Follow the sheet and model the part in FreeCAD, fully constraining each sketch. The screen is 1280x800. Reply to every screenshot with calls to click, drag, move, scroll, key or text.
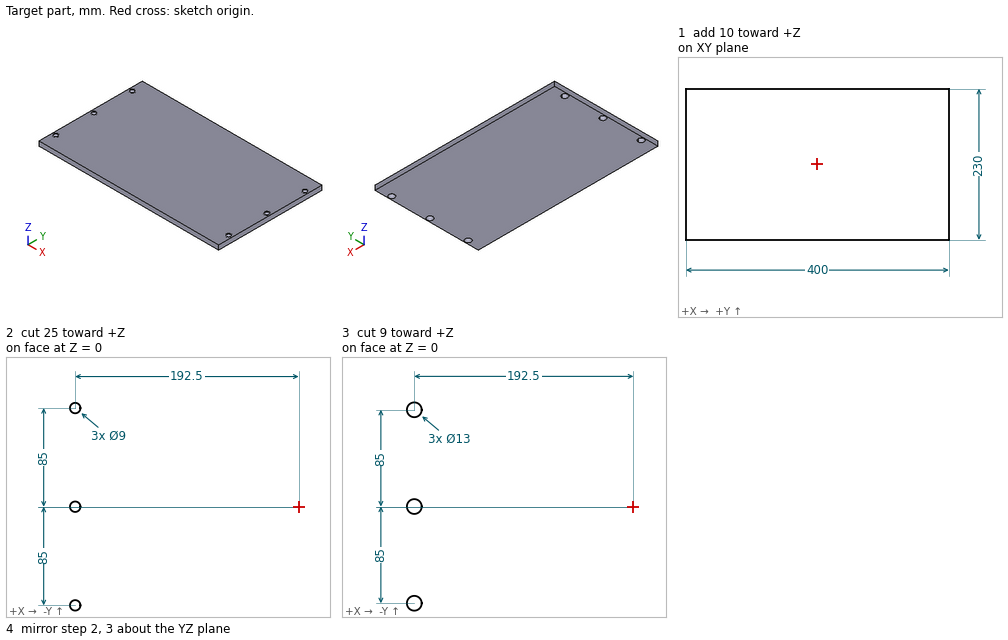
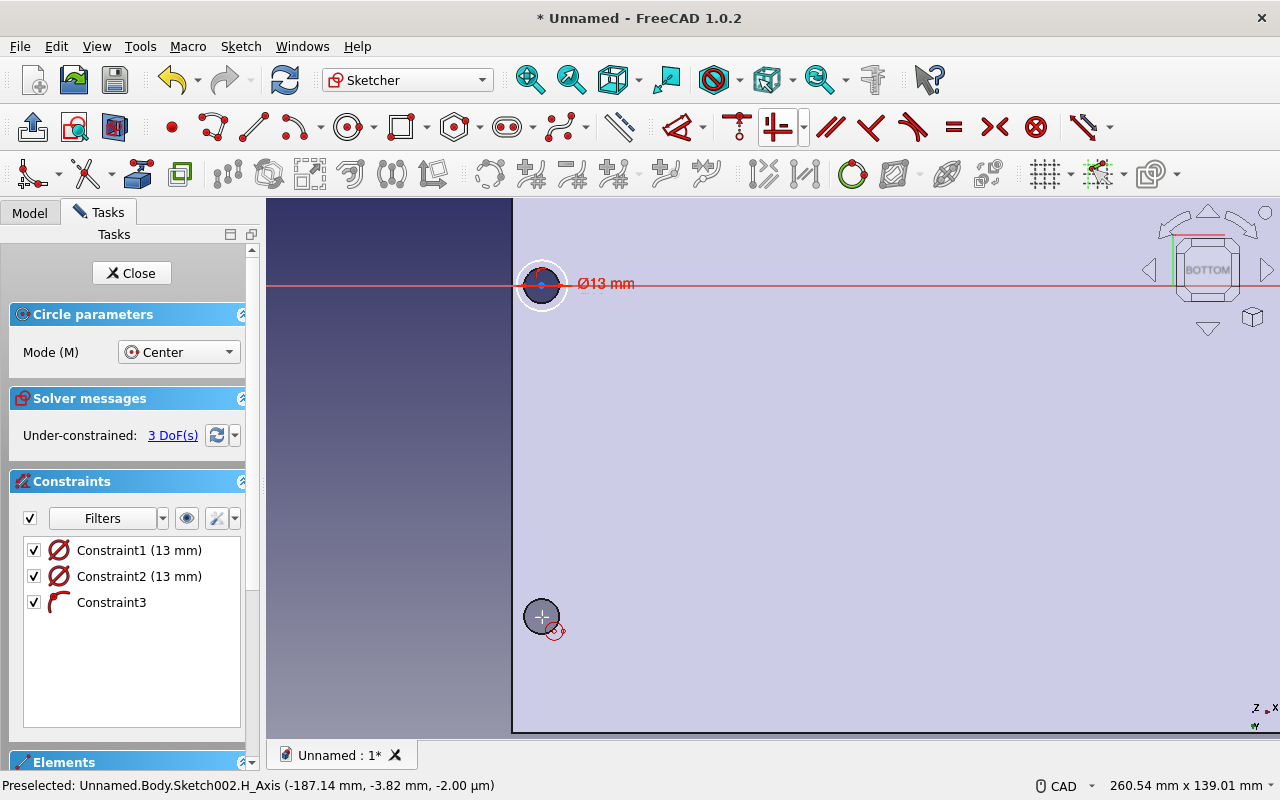
click(542, 616)
move(559, 599)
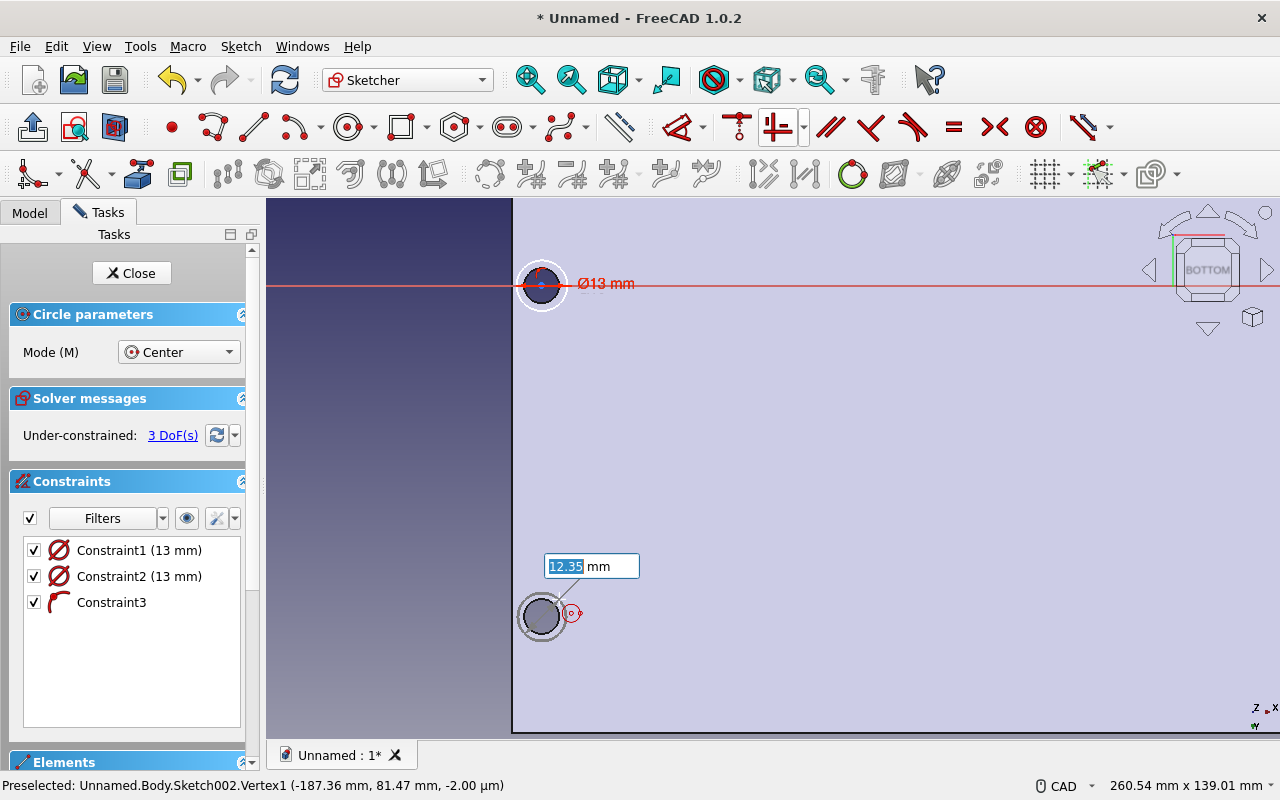
text(13)
key(Return)
key(Escape)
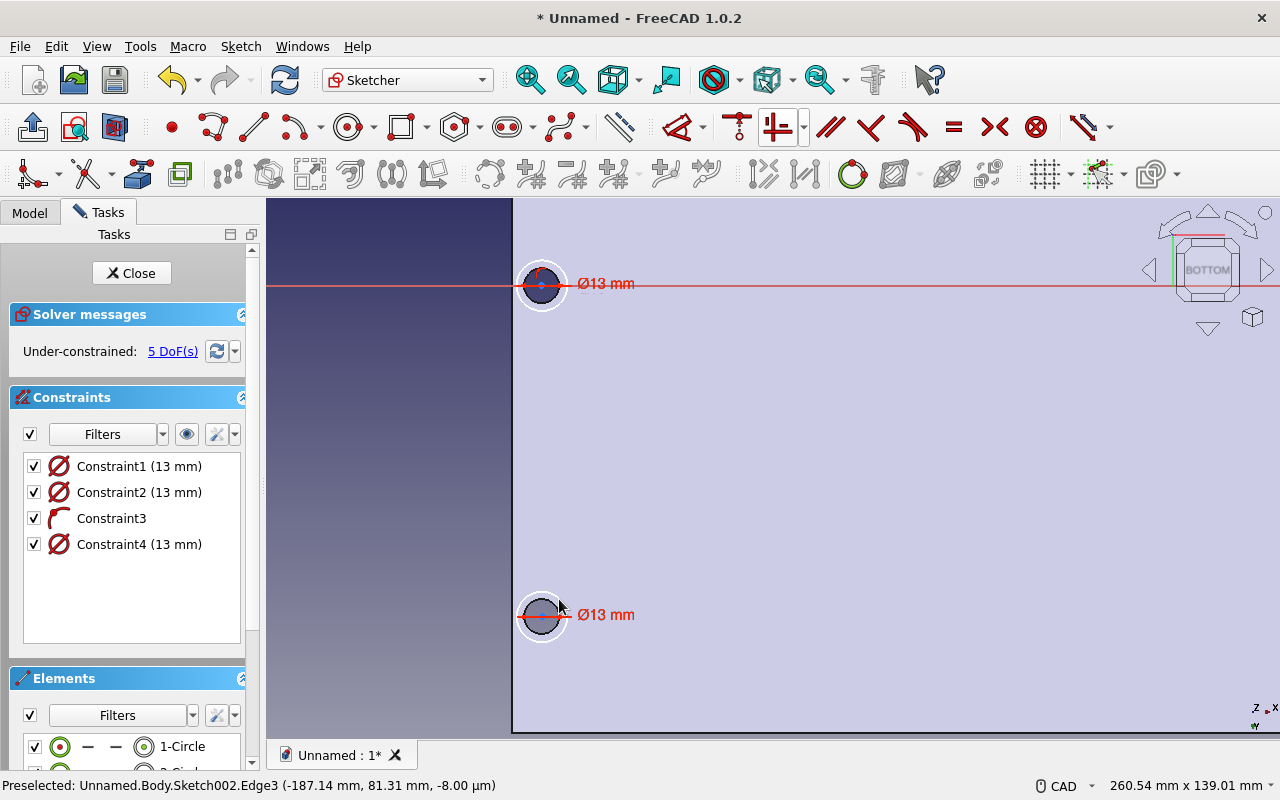
scroll(542, 618, down, 4)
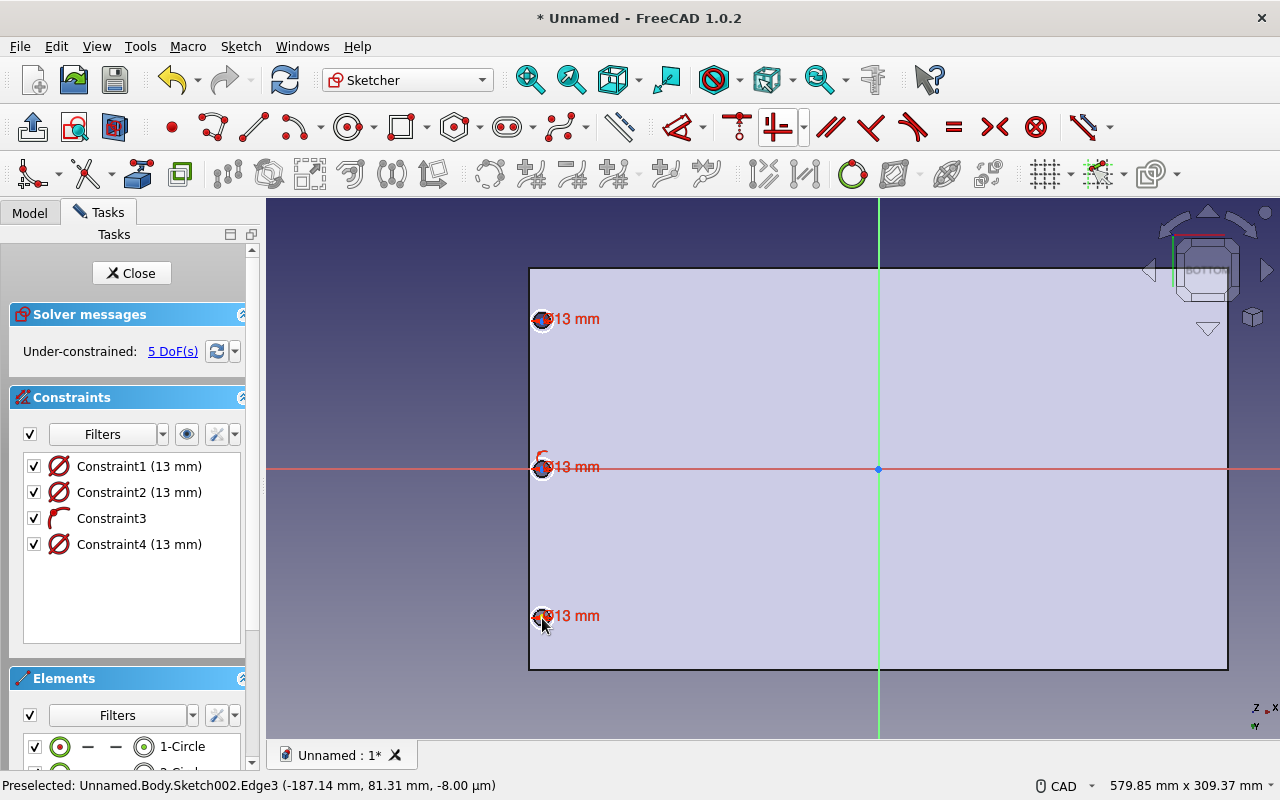
click(542, 321)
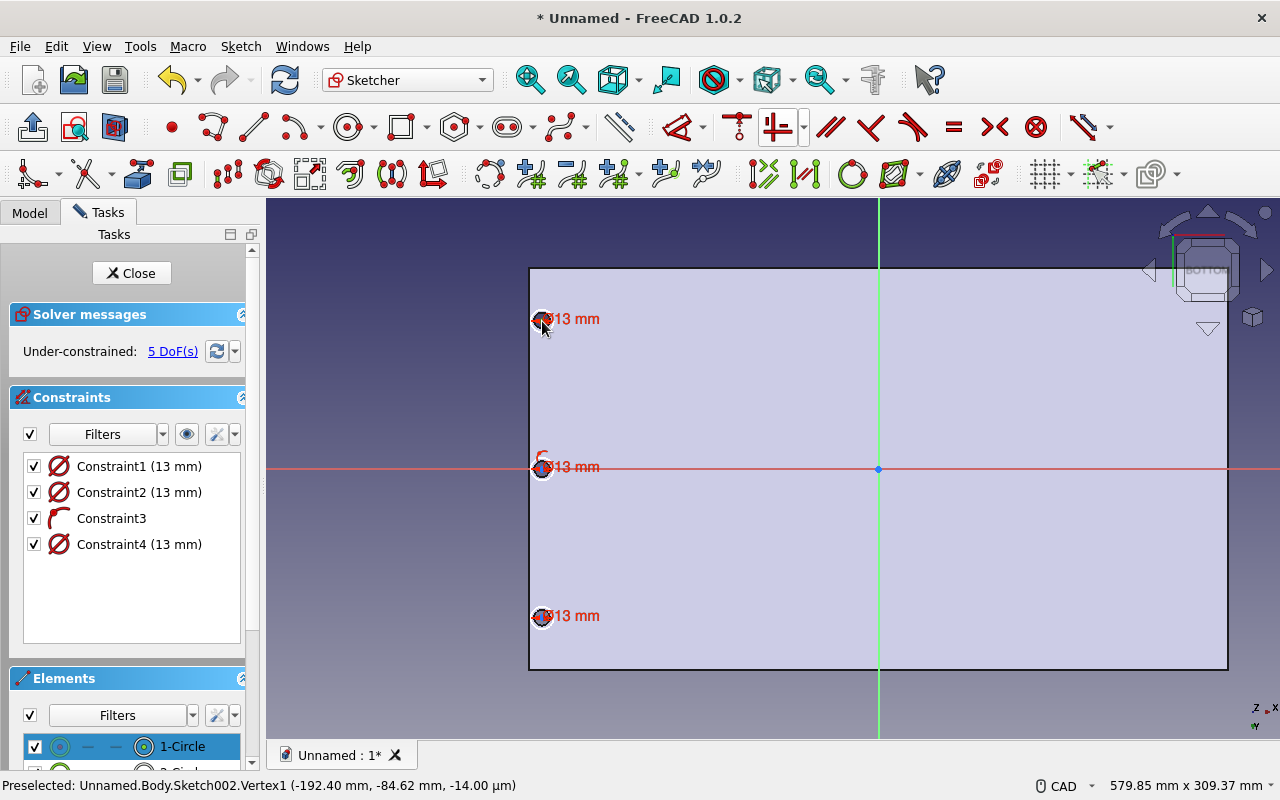
click(542, 469)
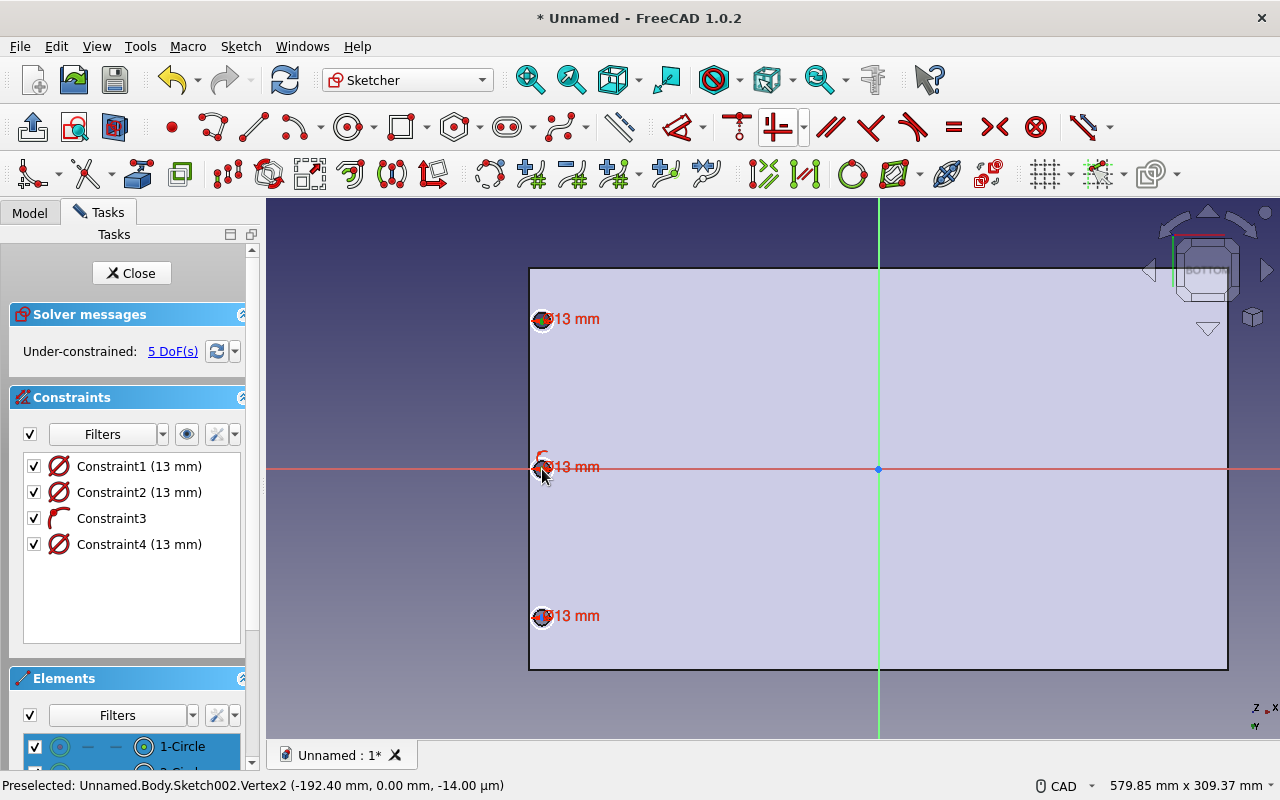
click(804, 128)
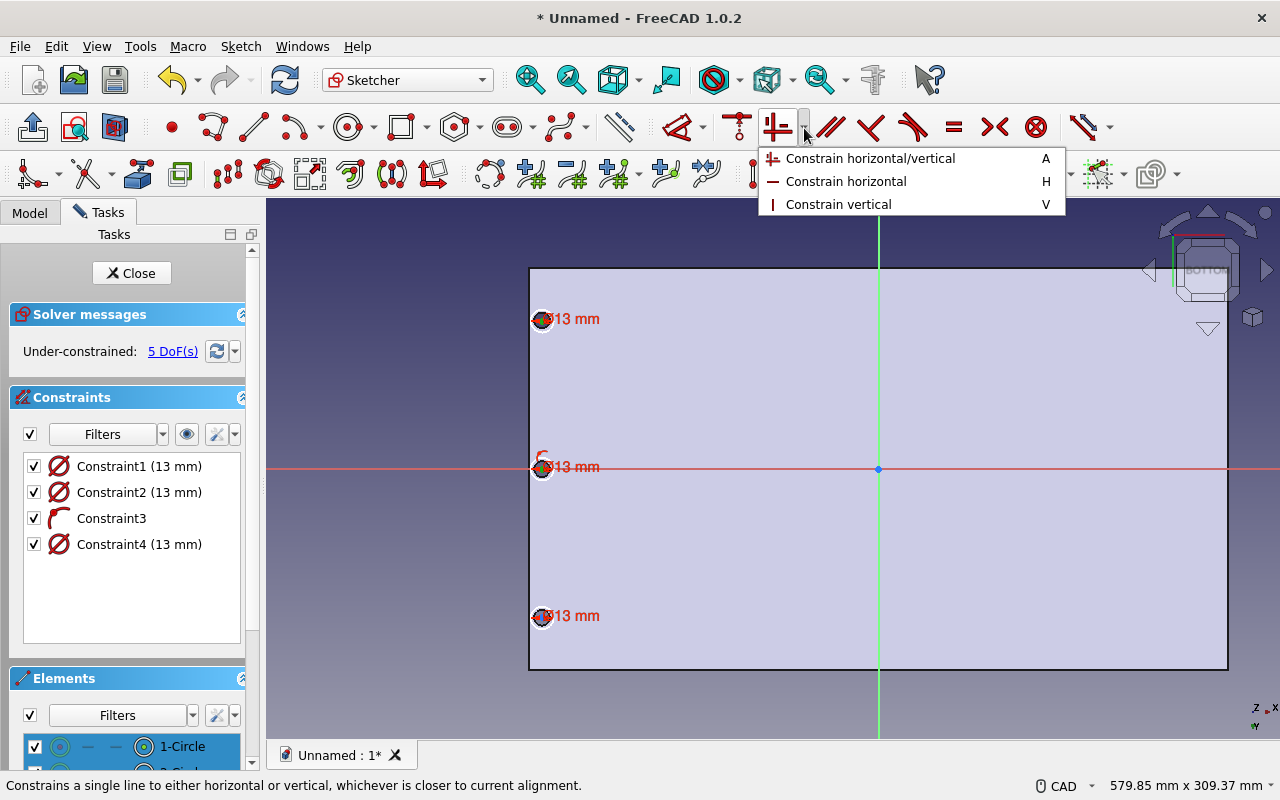
click(912, 204)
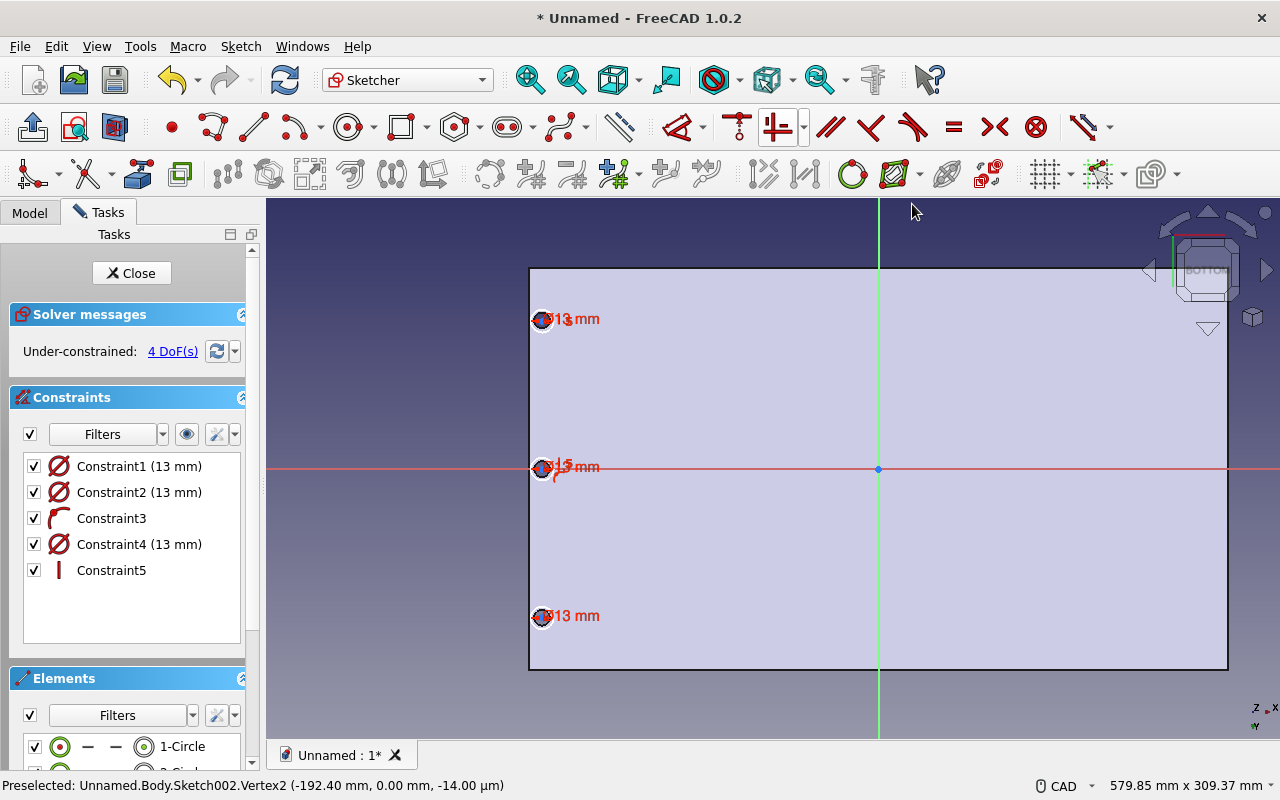
click(542, 469)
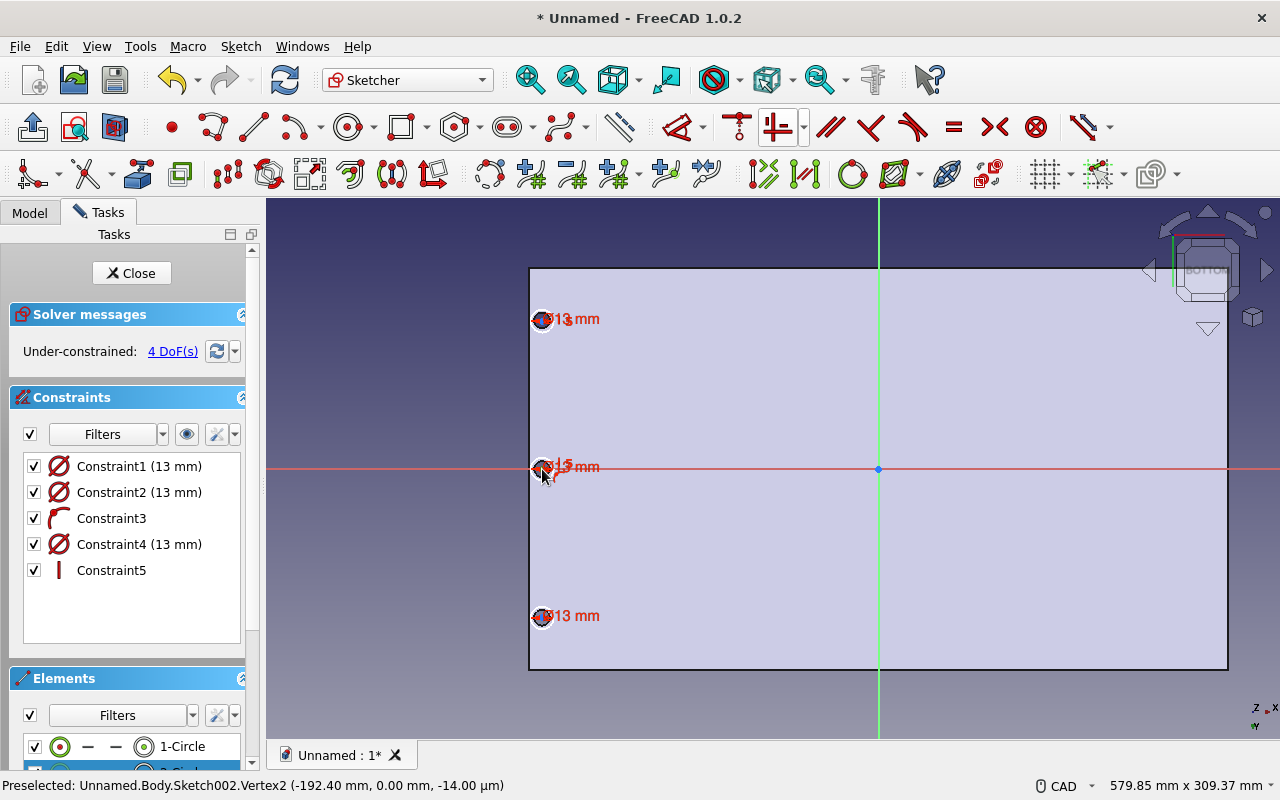
click(542, 618)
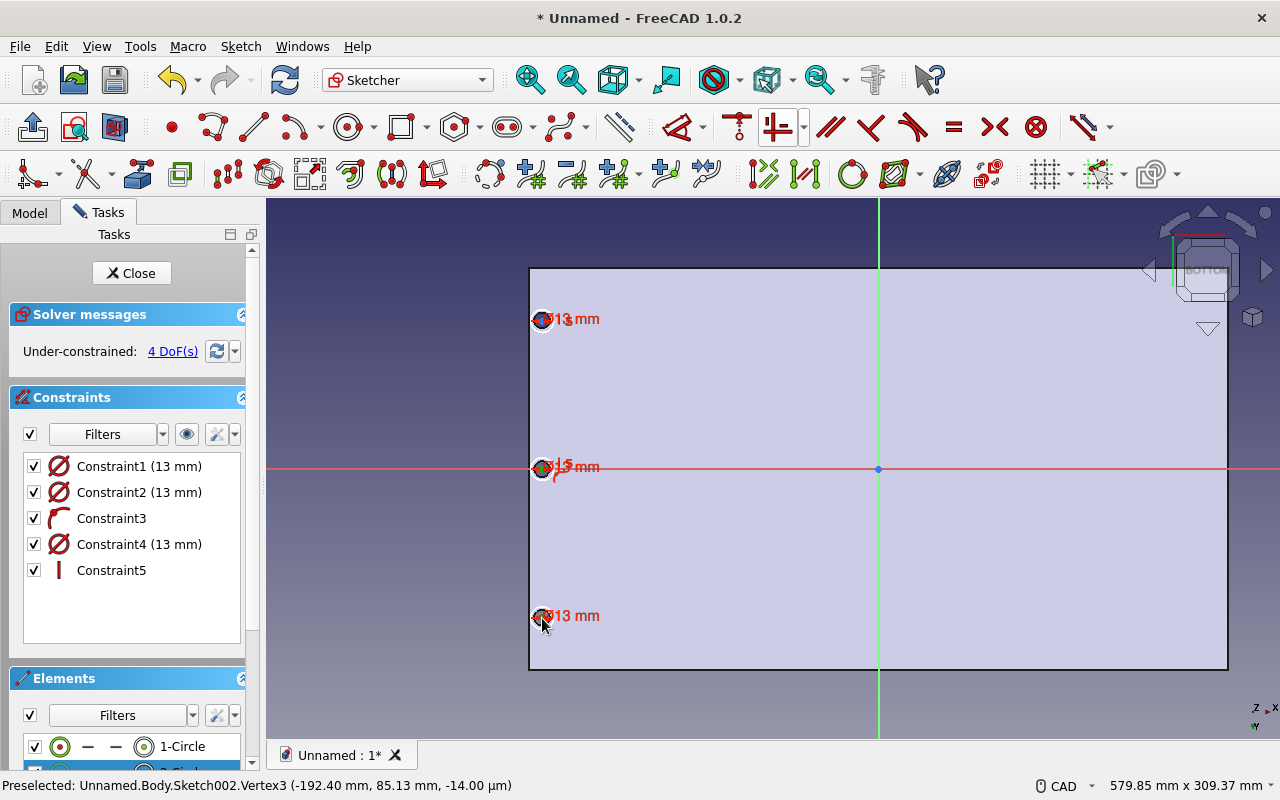
click(804, 128)